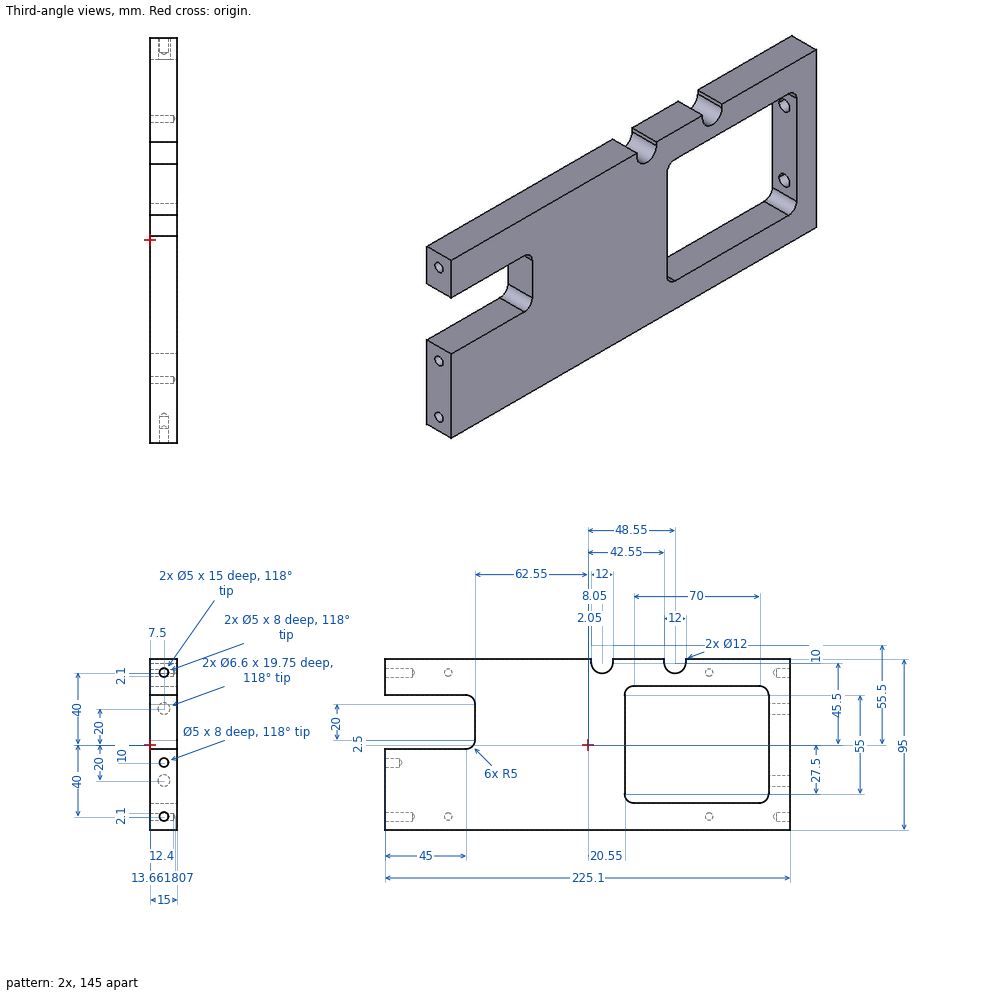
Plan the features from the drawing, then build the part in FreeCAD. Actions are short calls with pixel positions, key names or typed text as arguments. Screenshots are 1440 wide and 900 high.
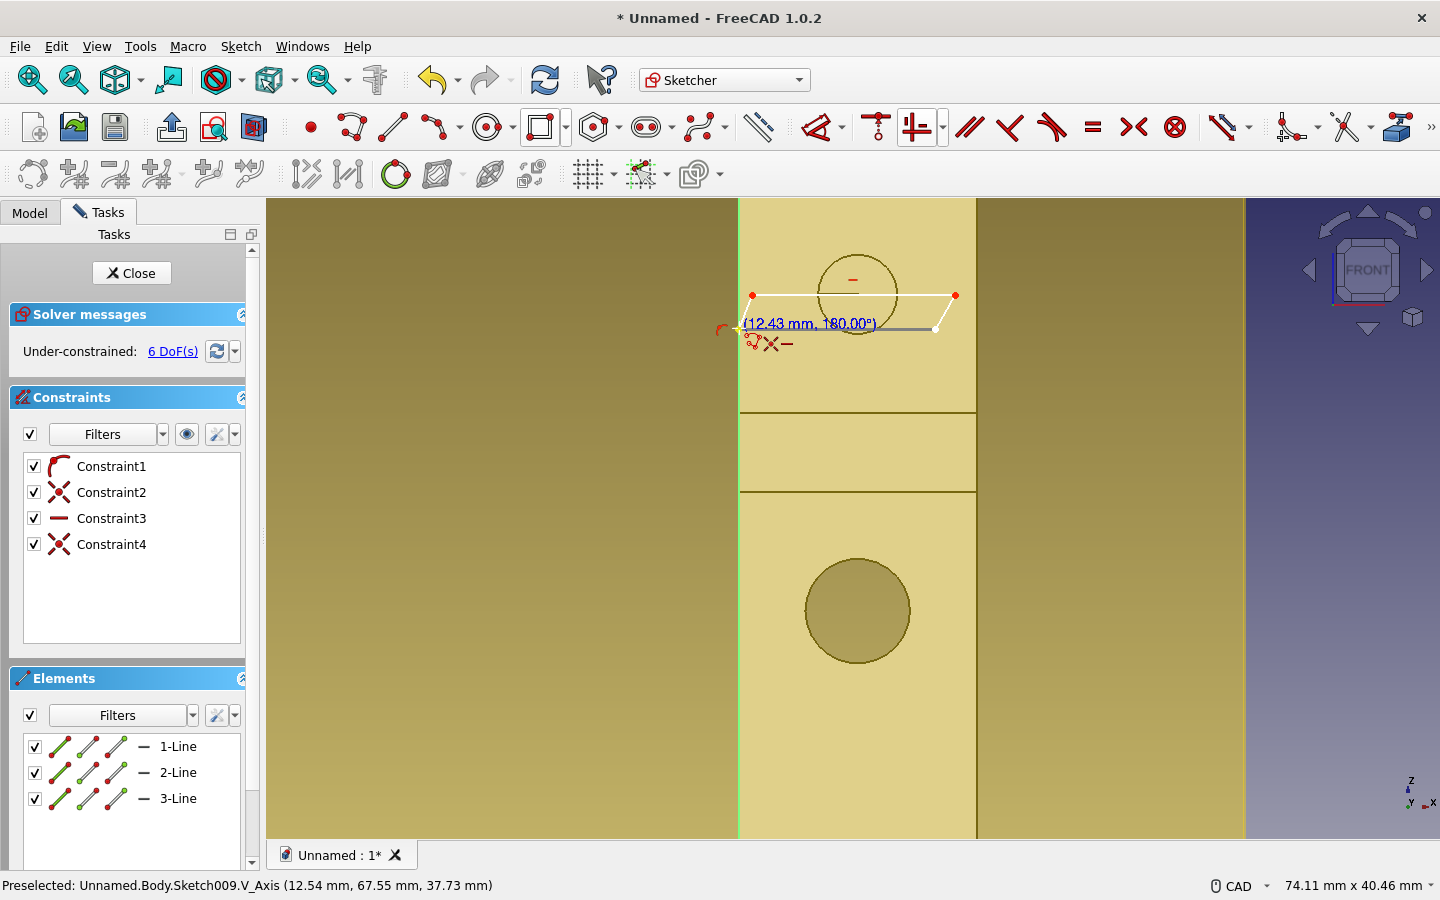
click(739, 329)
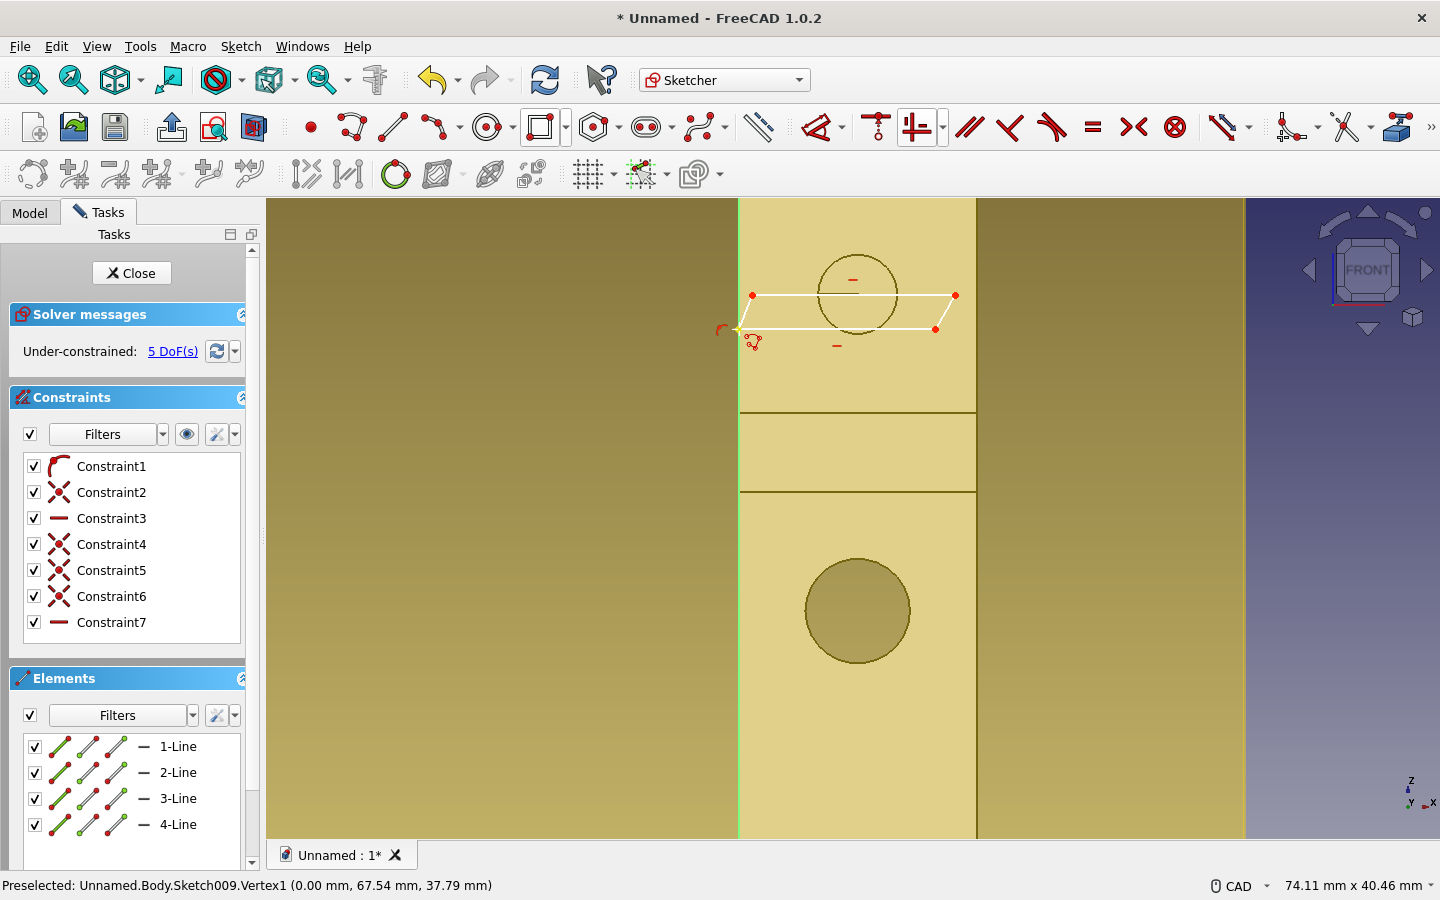
click(393, 128)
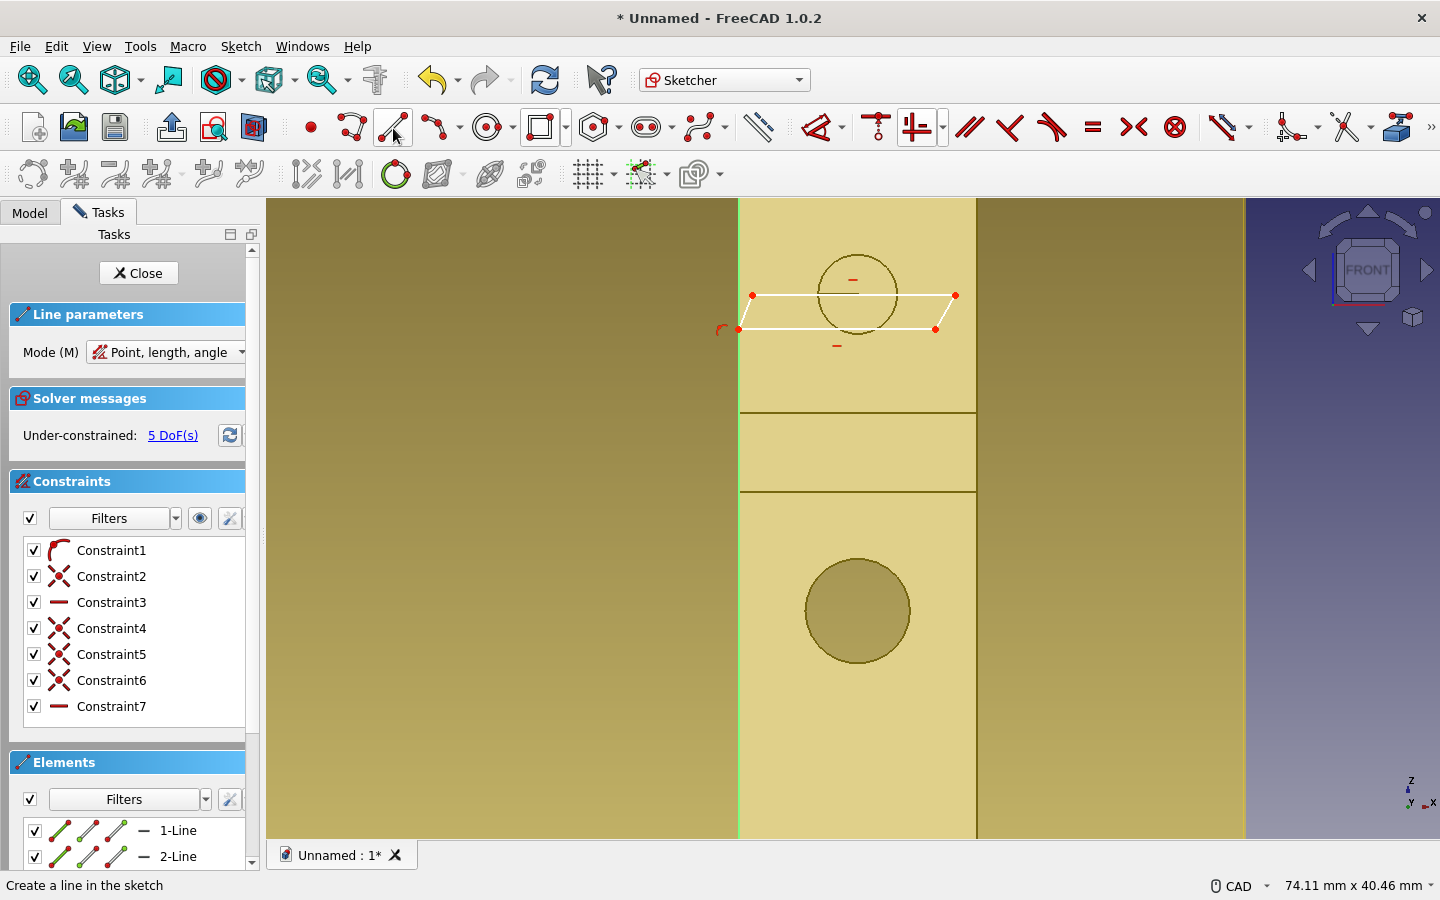
click(717, 294)
click(652, 294)
key(Escape)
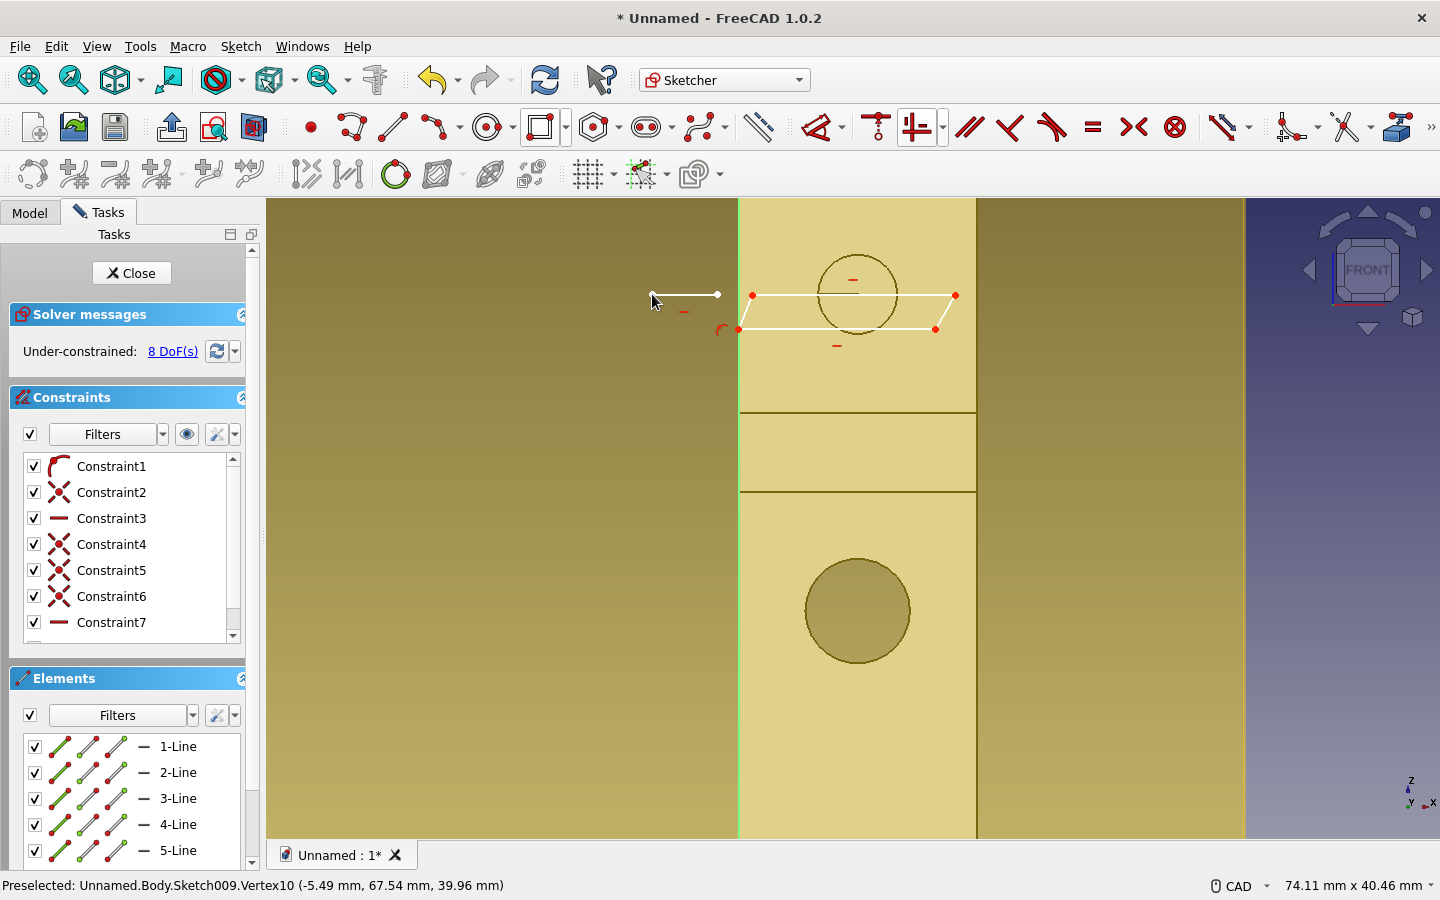
click(698, 295)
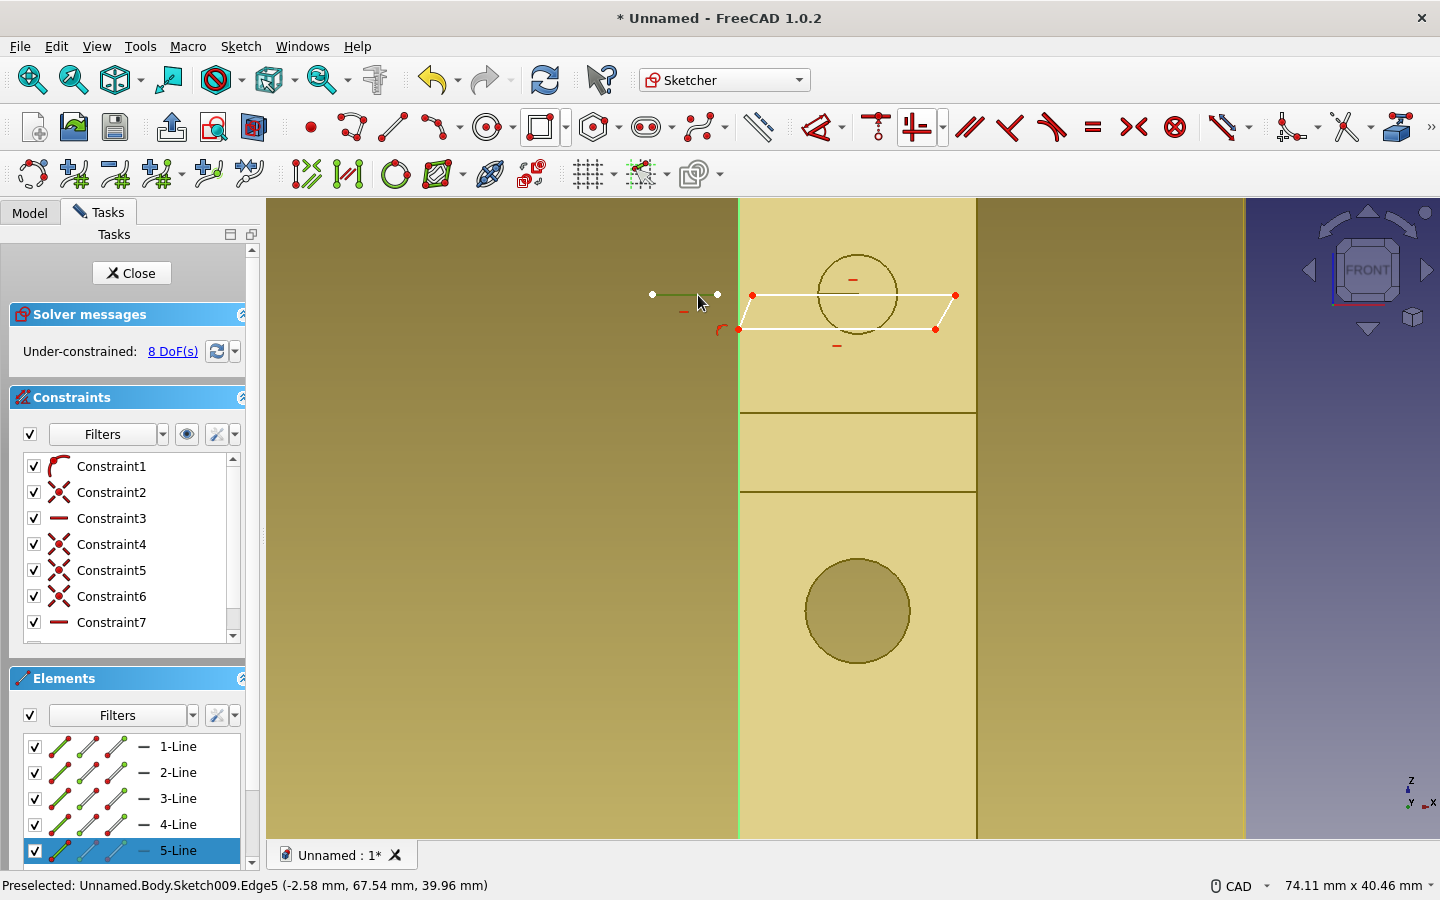
click(759, 128)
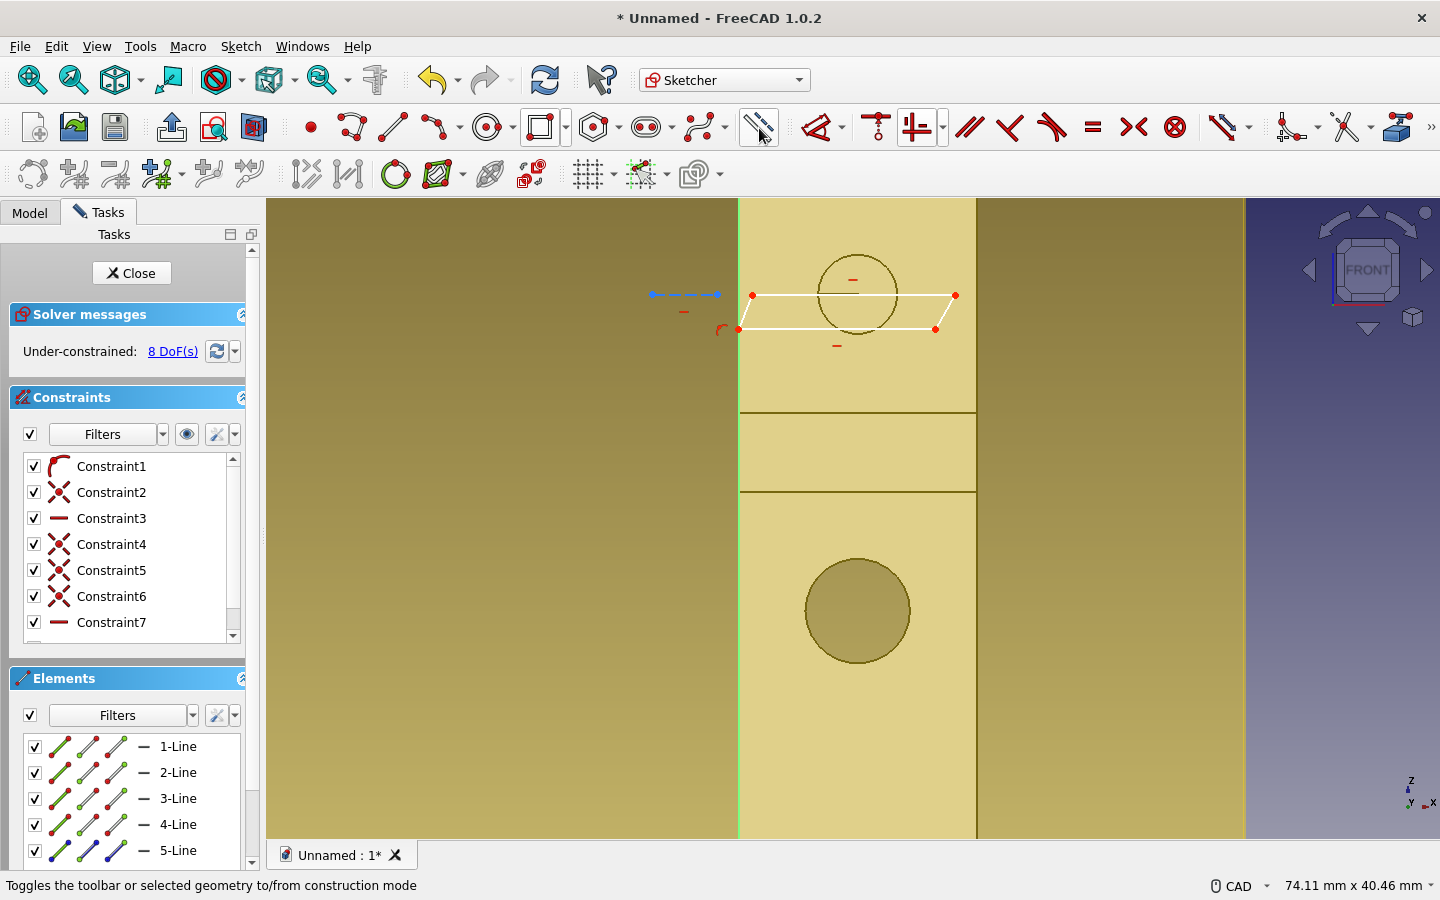
scroll(748, 305, up, 2)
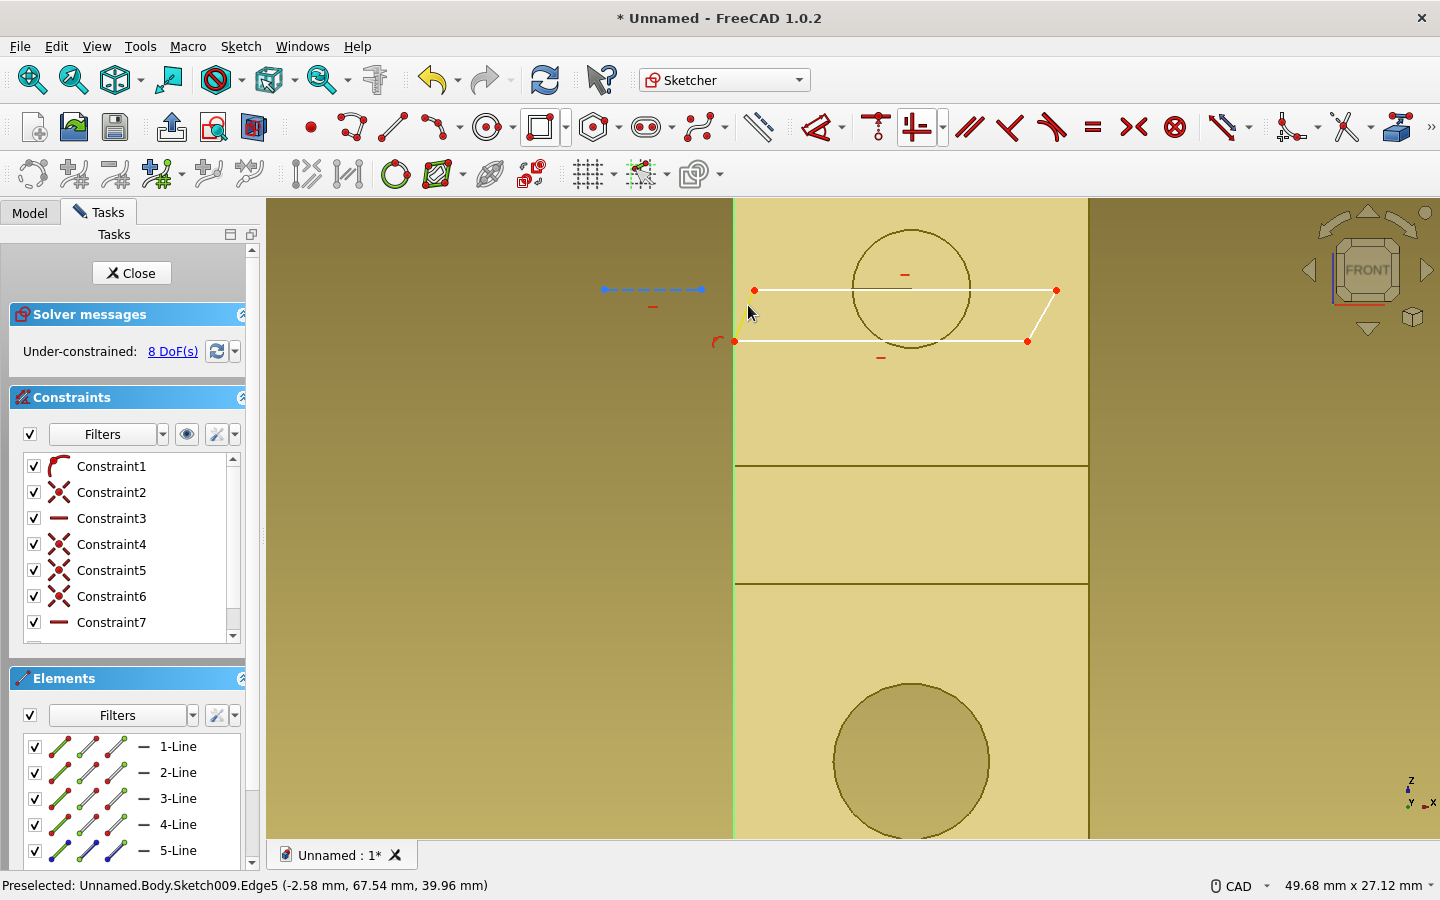
click(748, 305)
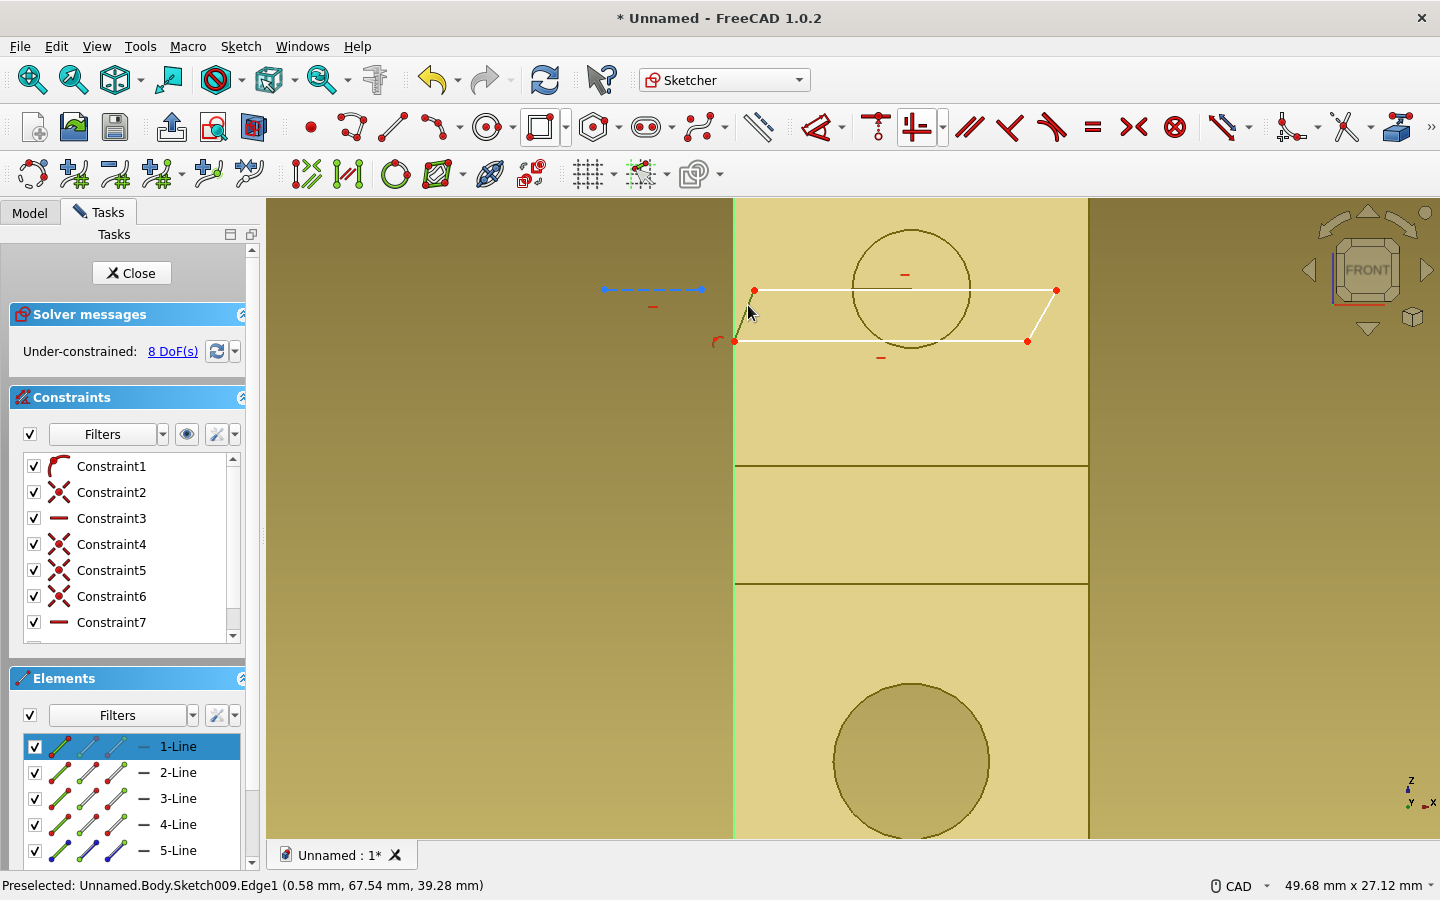
key(v)